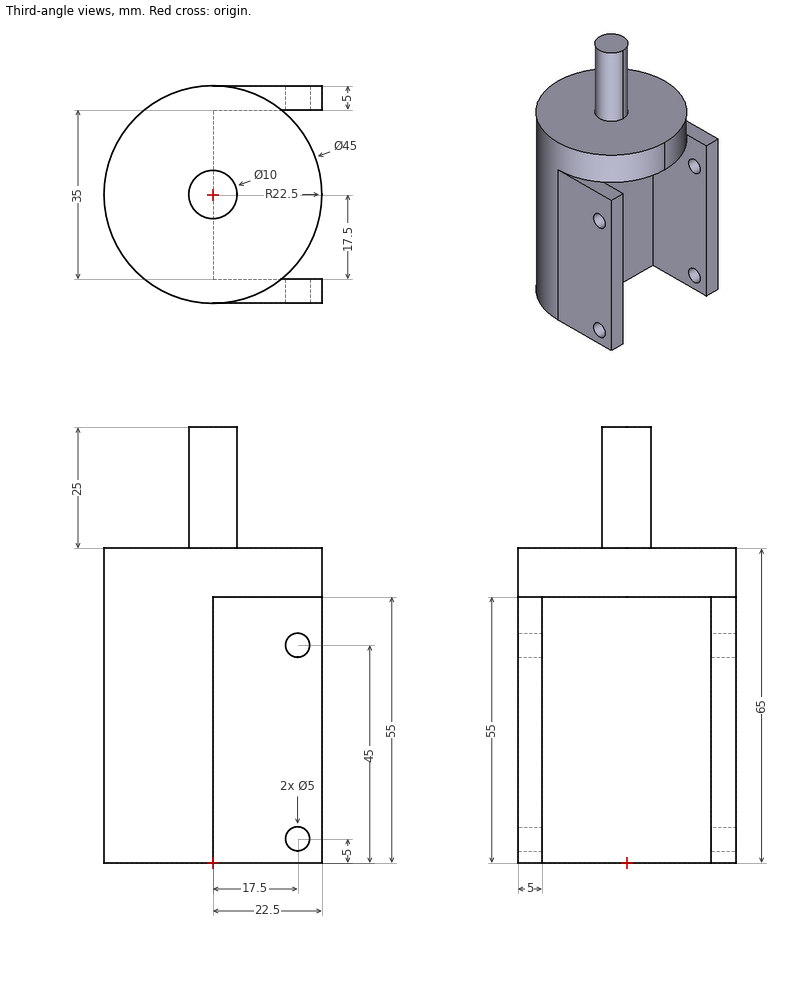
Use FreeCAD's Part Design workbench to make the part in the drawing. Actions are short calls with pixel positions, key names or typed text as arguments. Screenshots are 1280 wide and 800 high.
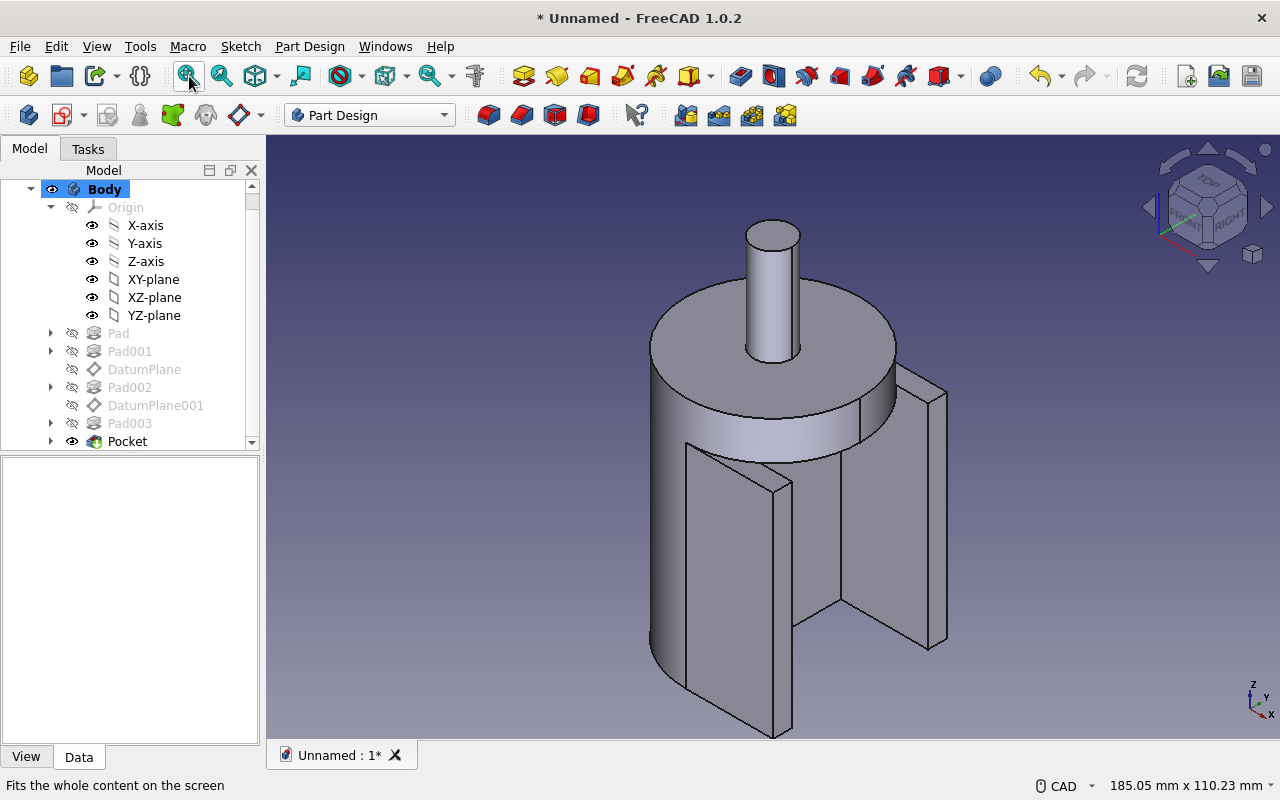
click(189, 76)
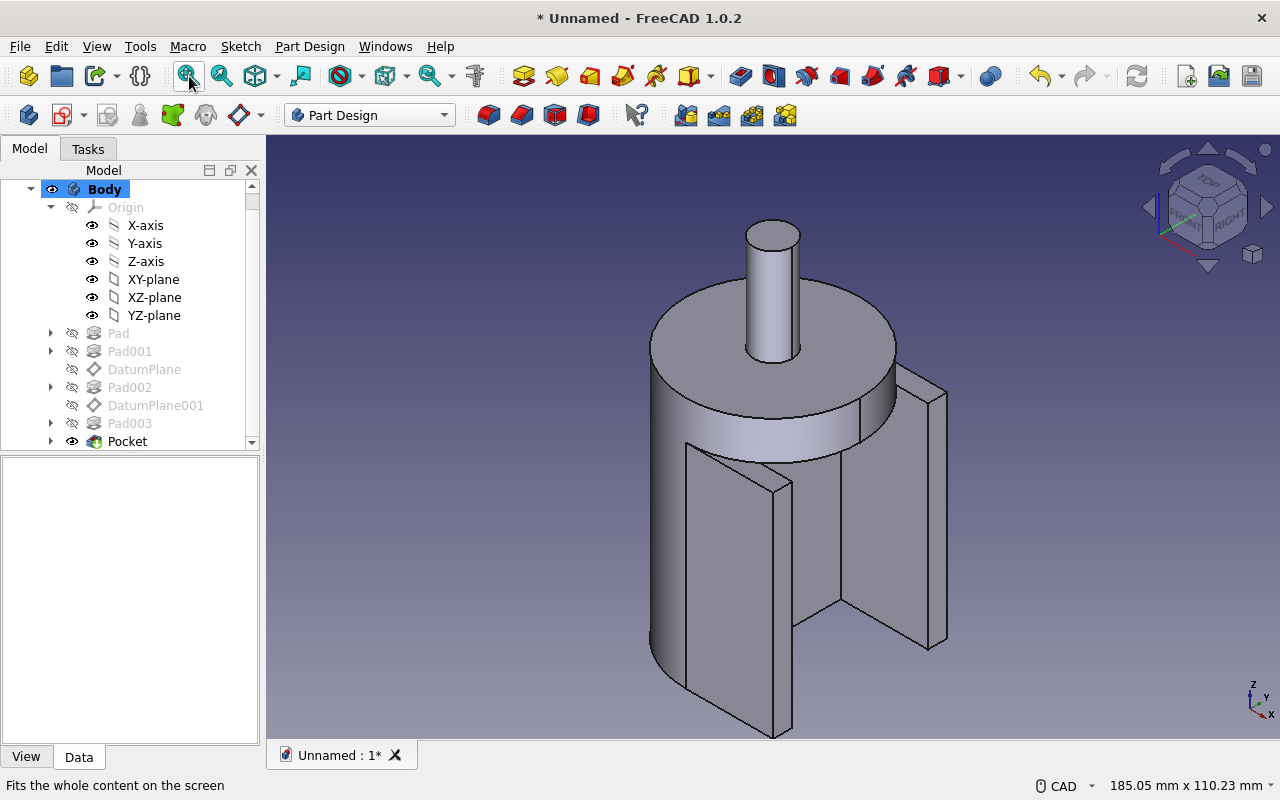
click(729, 519)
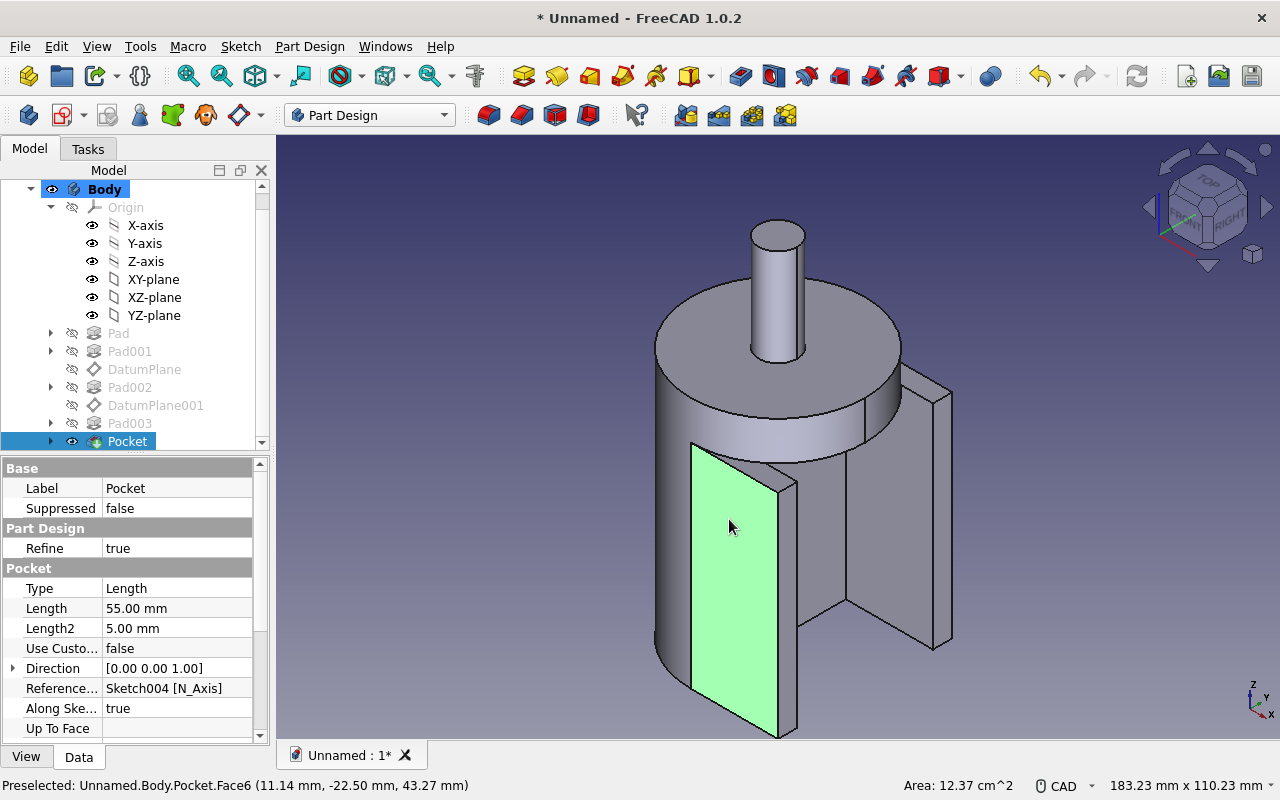
click(62, 116)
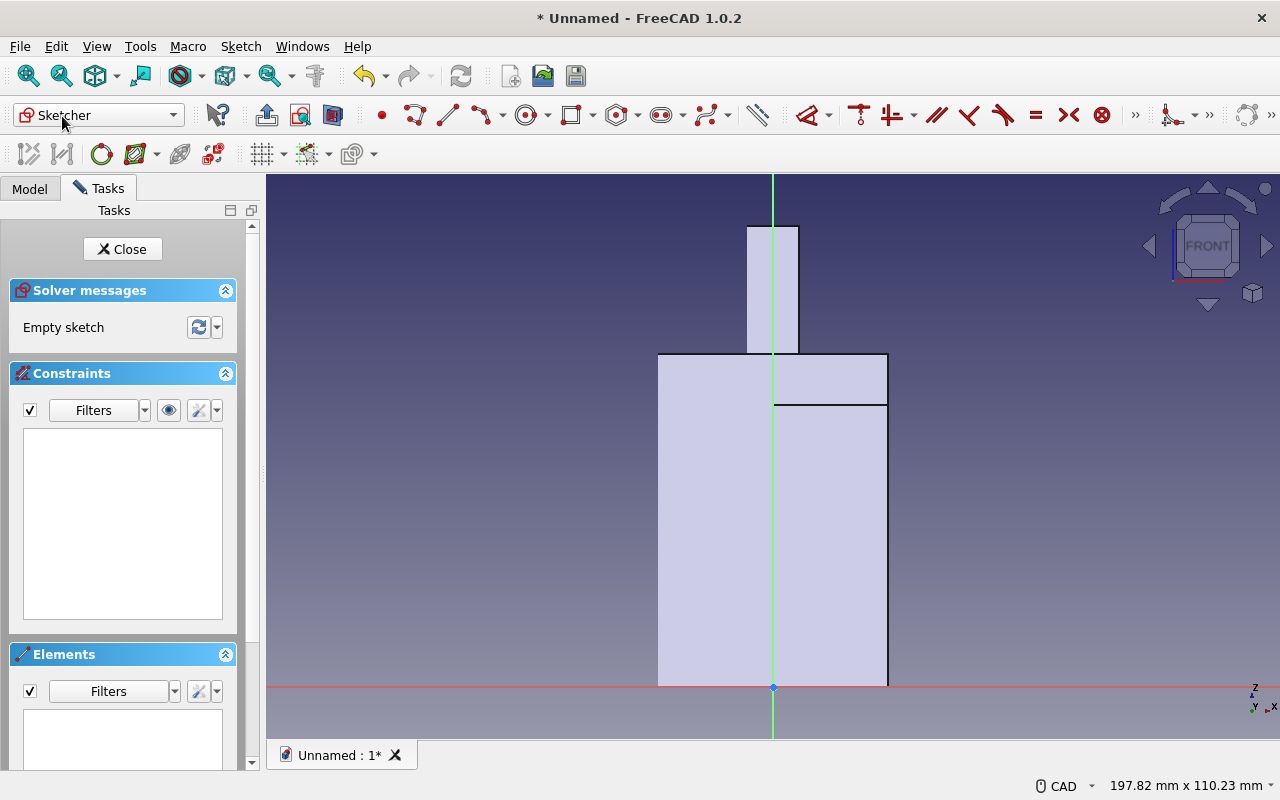
scroll(1068, 711, up, 2)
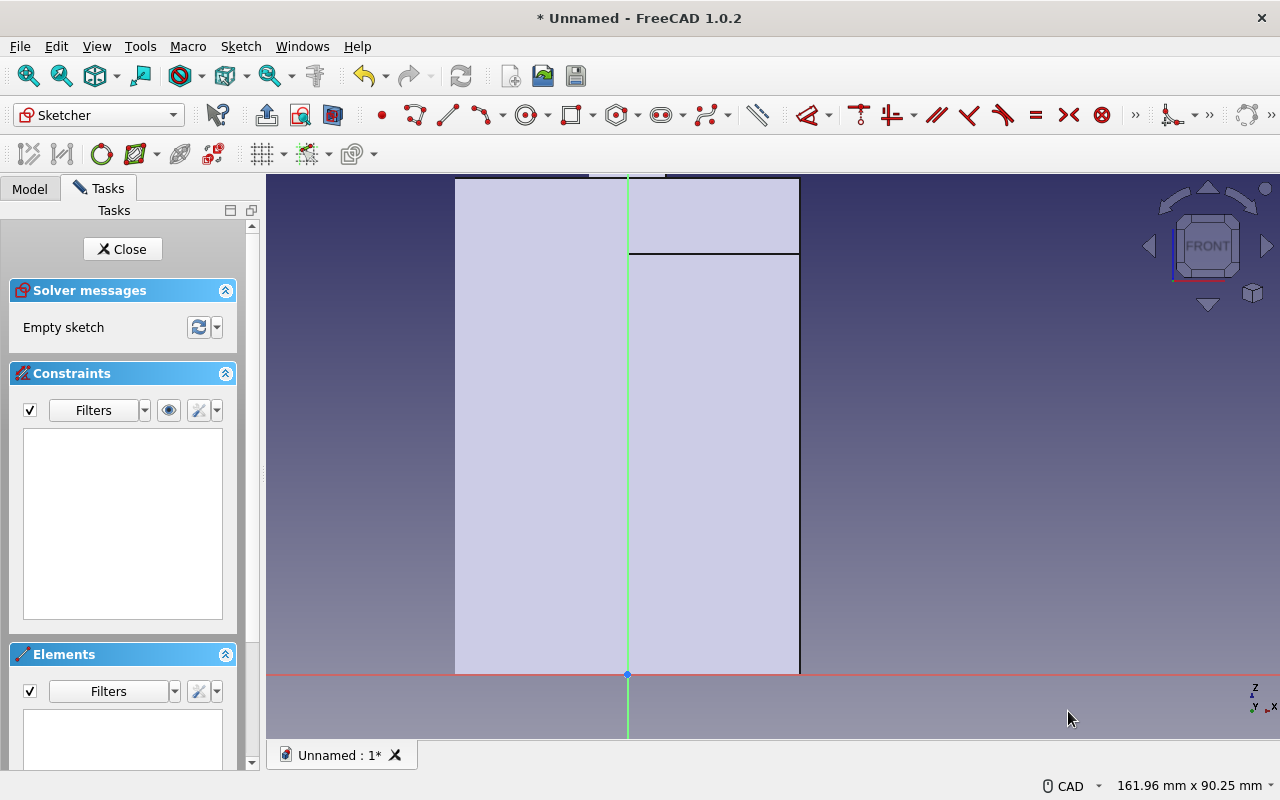
click(526, 116)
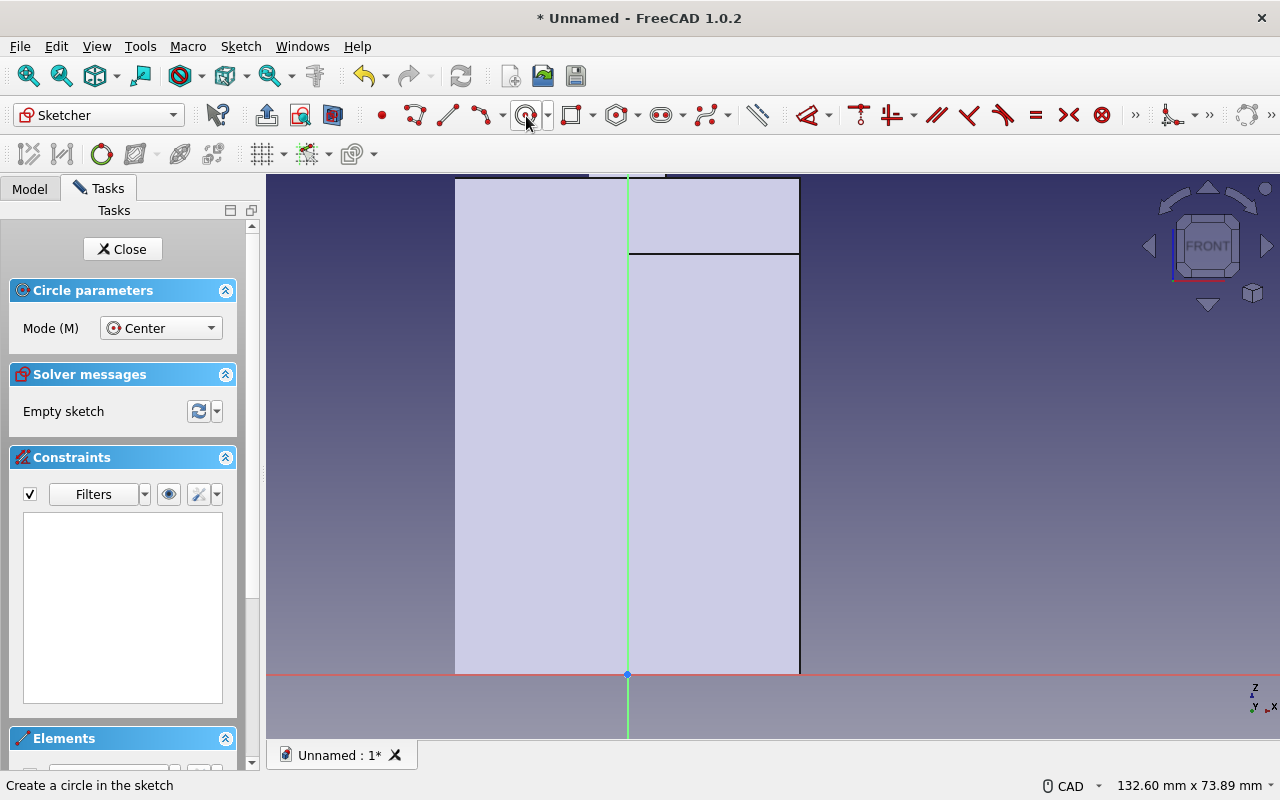
click(761, 637)
click(775, 623)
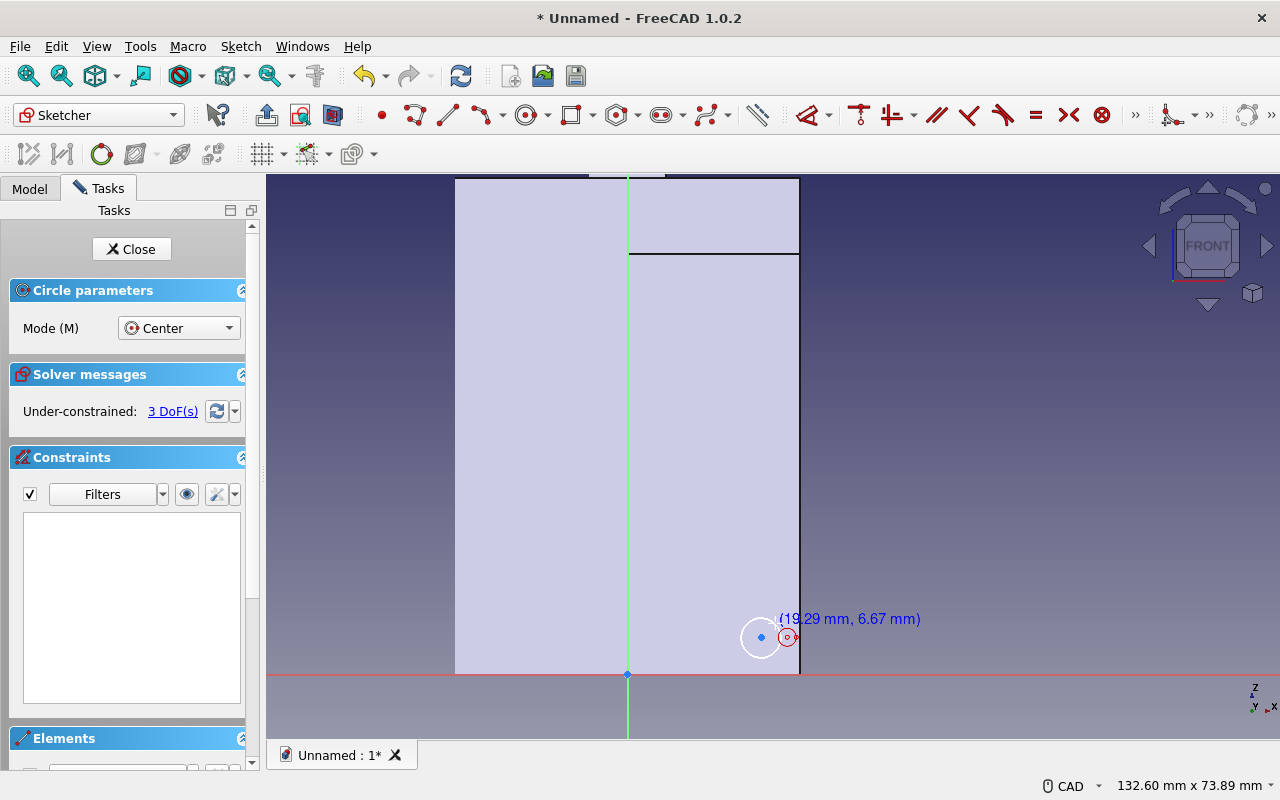
click(761, 331)
click(775, 317)
key(Escape)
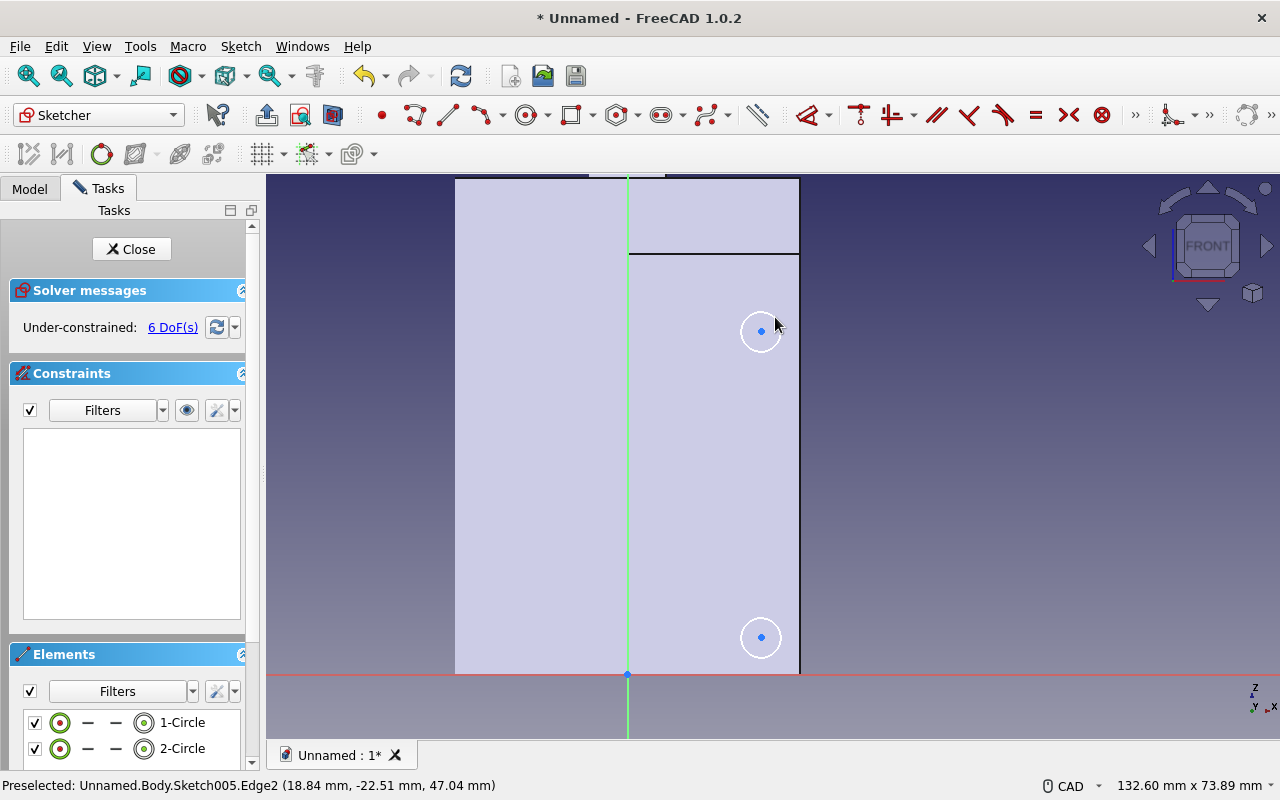
click(775, 624)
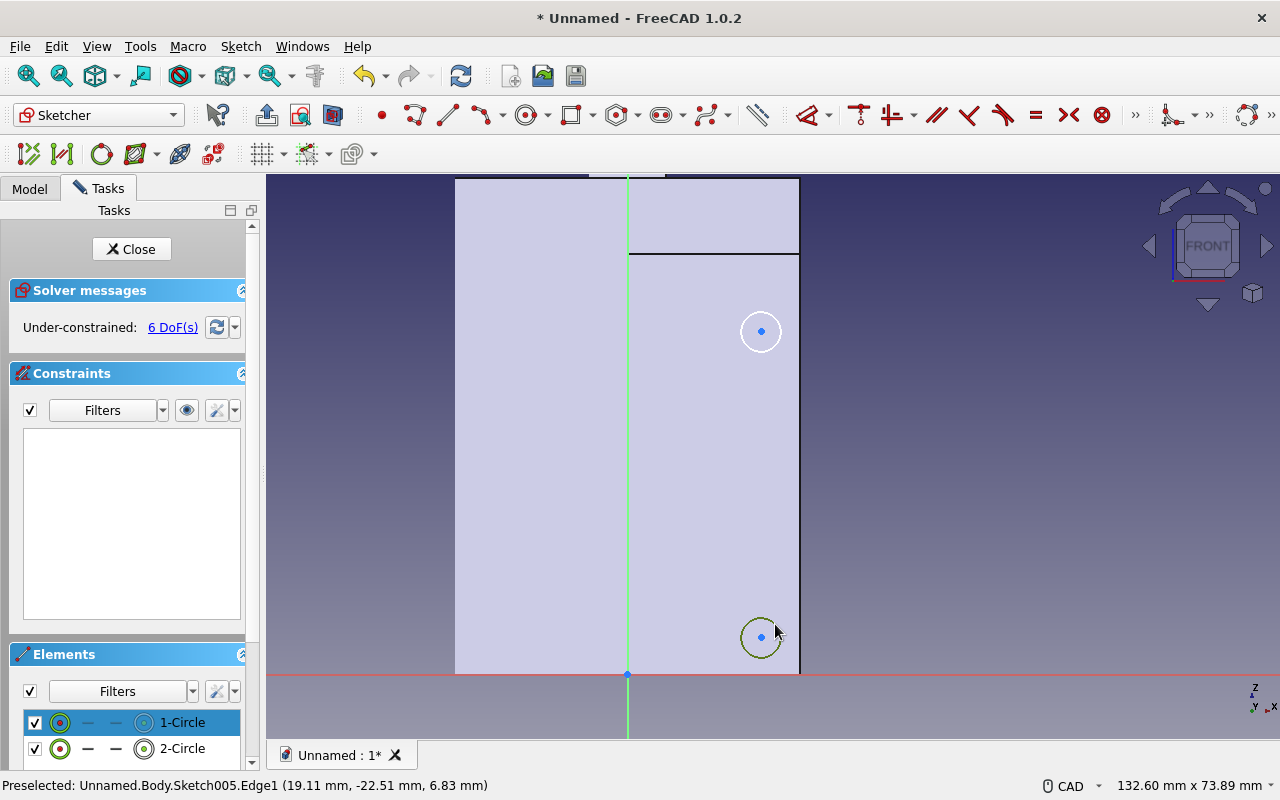
click(775, 318)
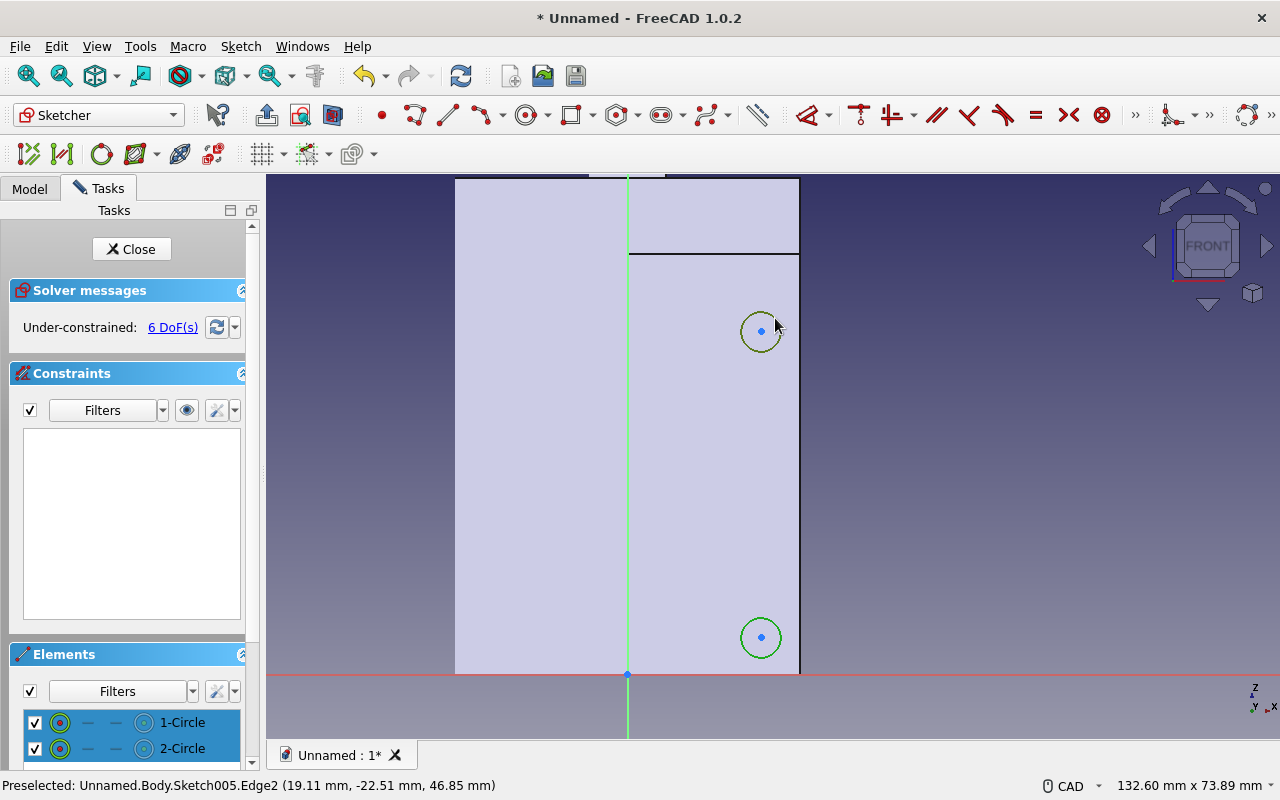
click(1036, 116)